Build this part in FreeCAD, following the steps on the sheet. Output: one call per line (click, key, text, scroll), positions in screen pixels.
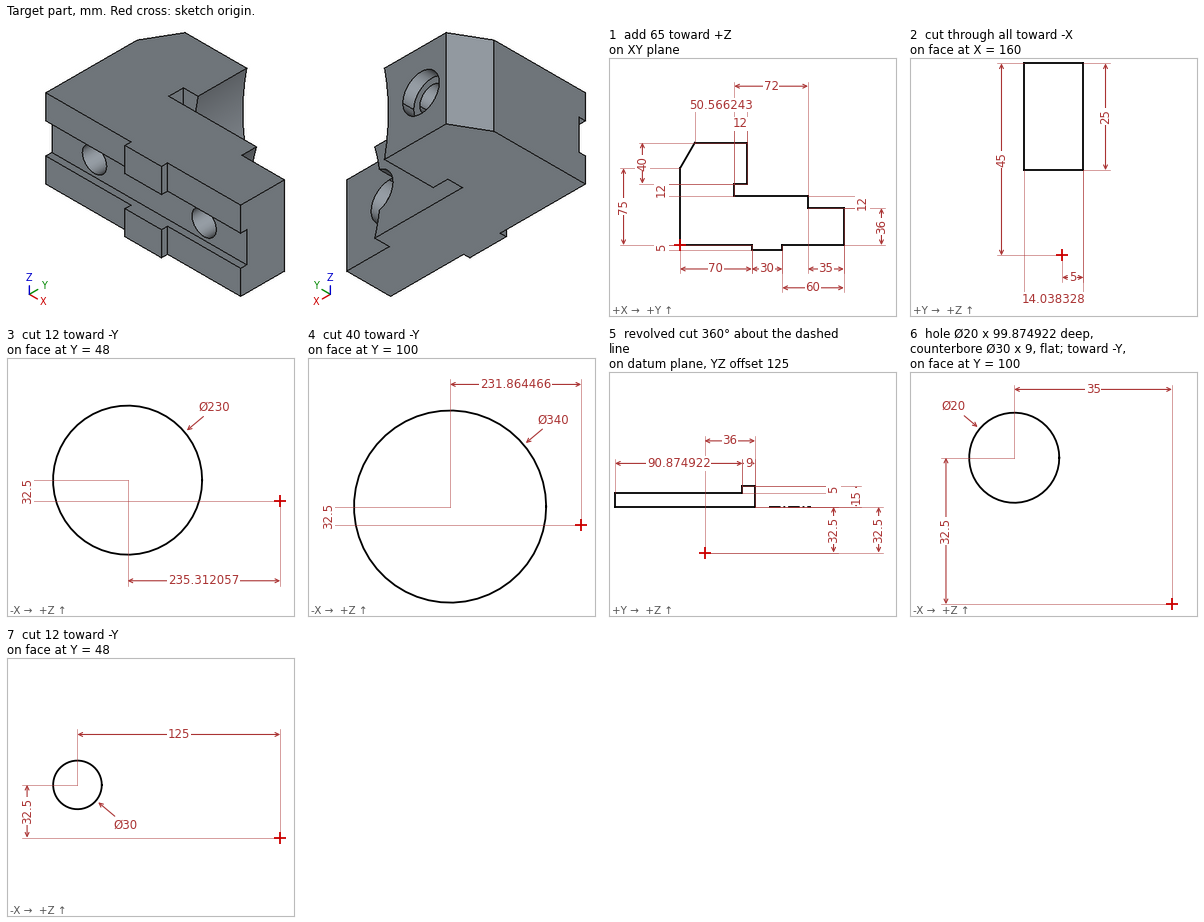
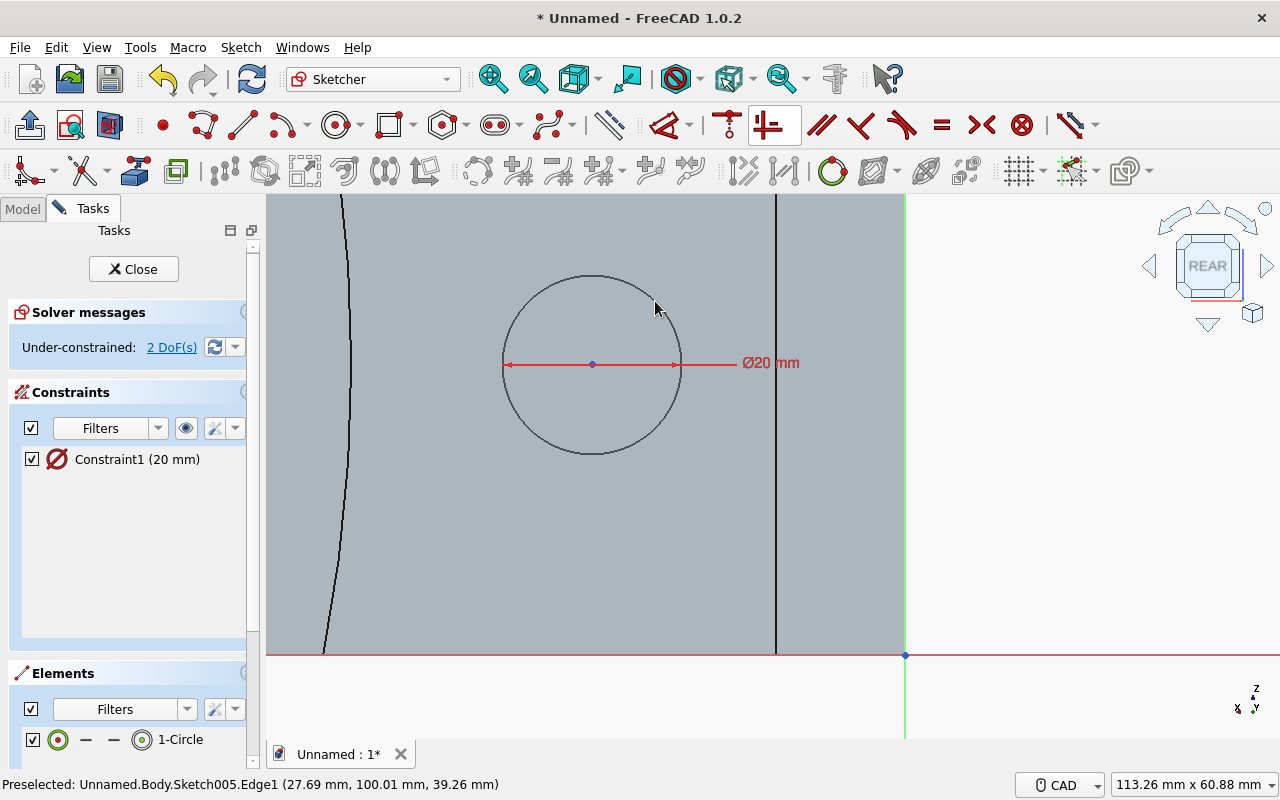
key(d)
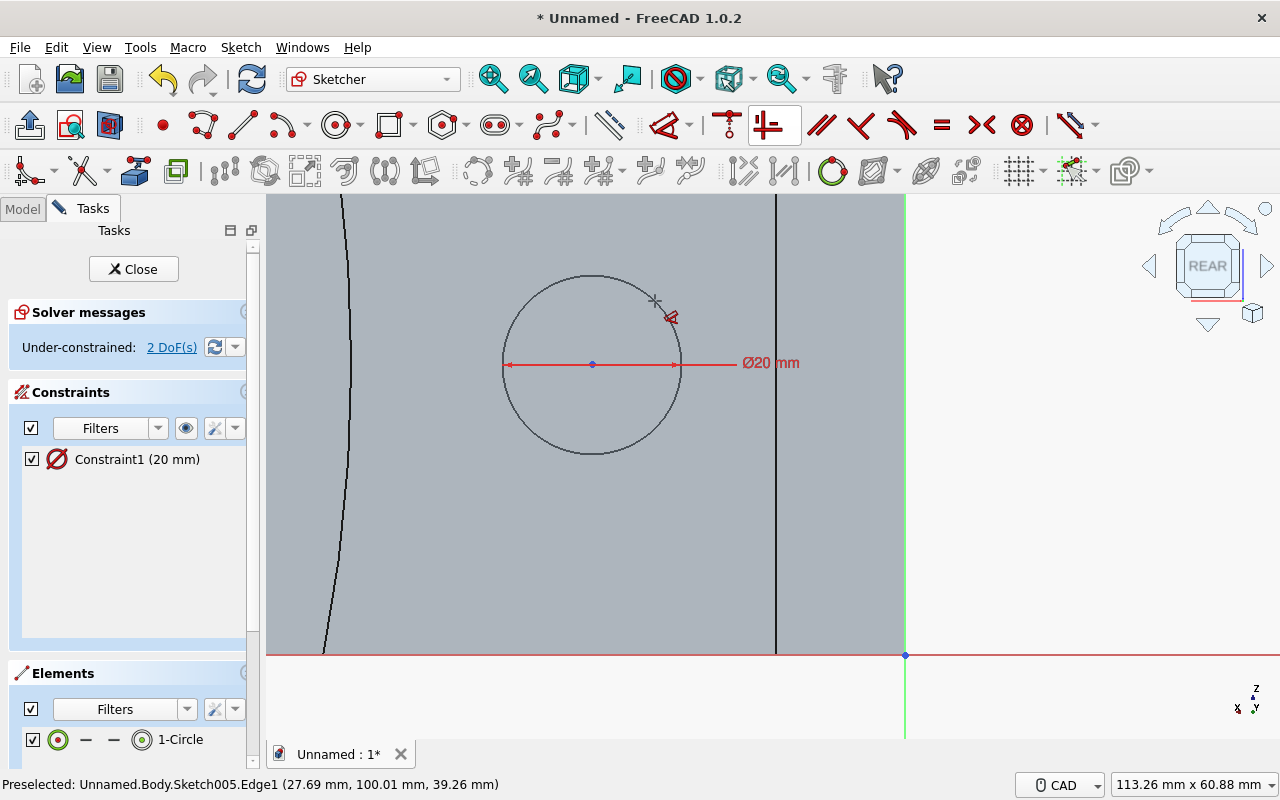
click(592, 365)
click(749, 689)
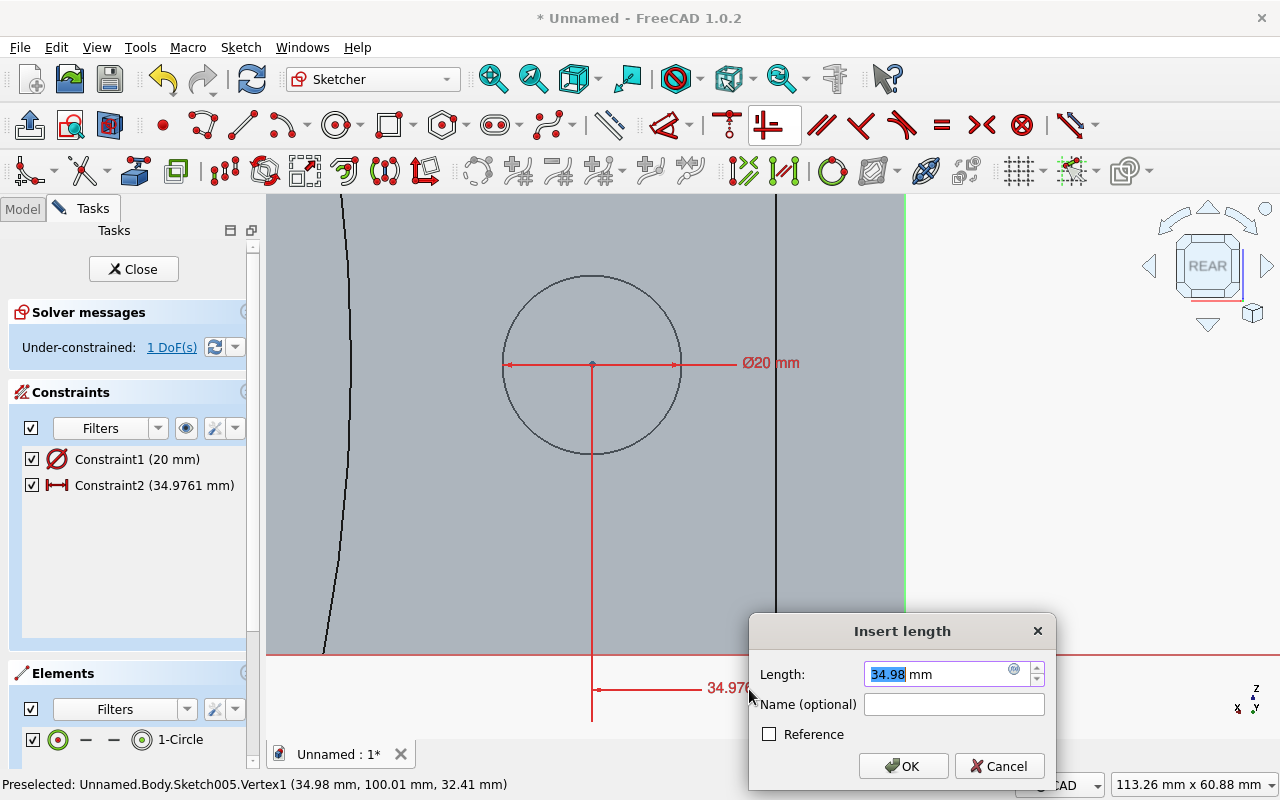
text(35)
key(Return)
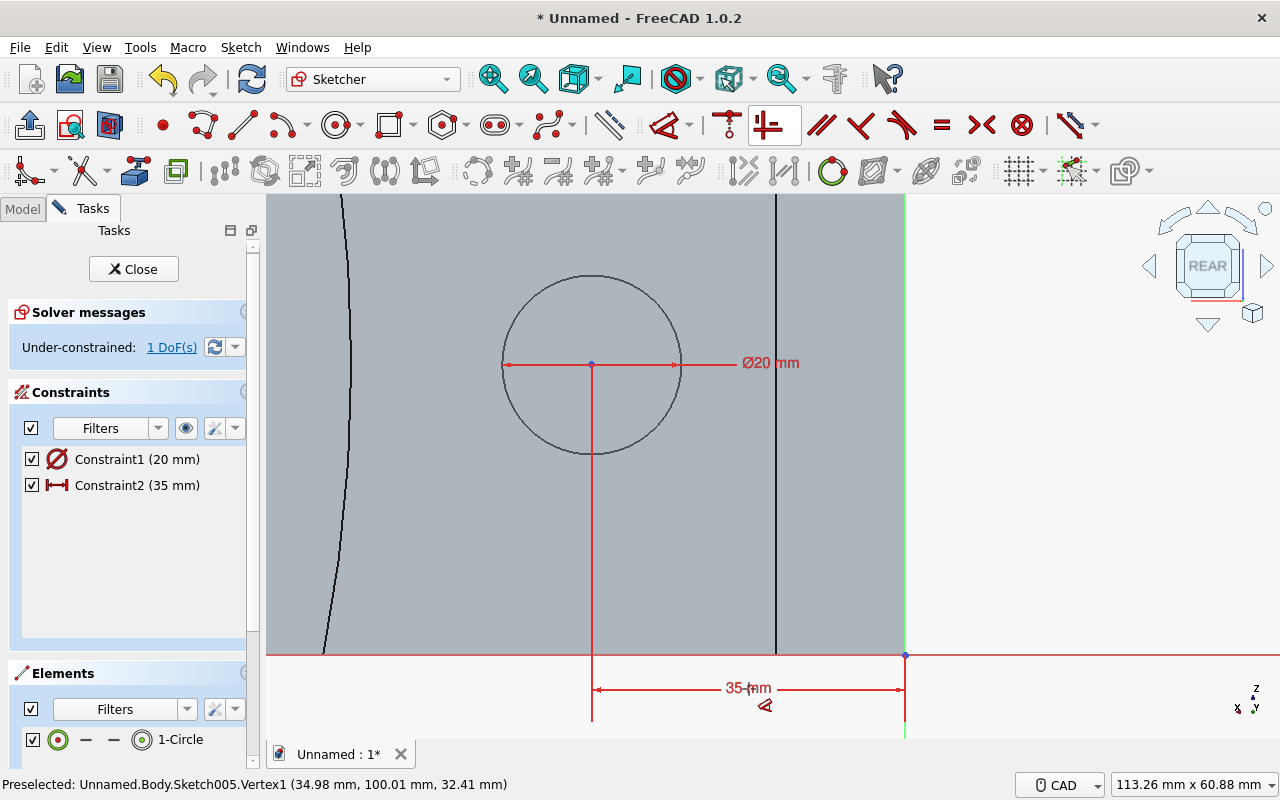
click(592, 365)
click(939, 510)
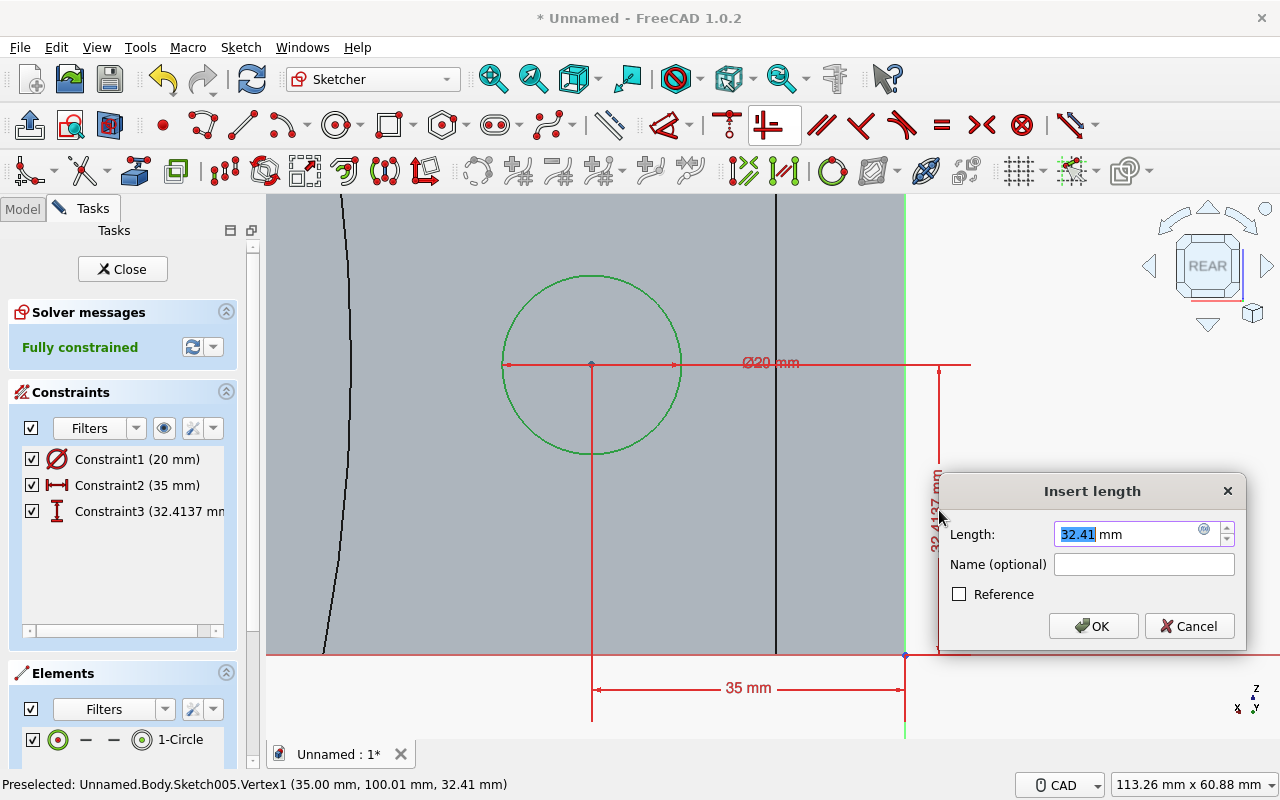
text(32.5)
key(Return)
key(Escape)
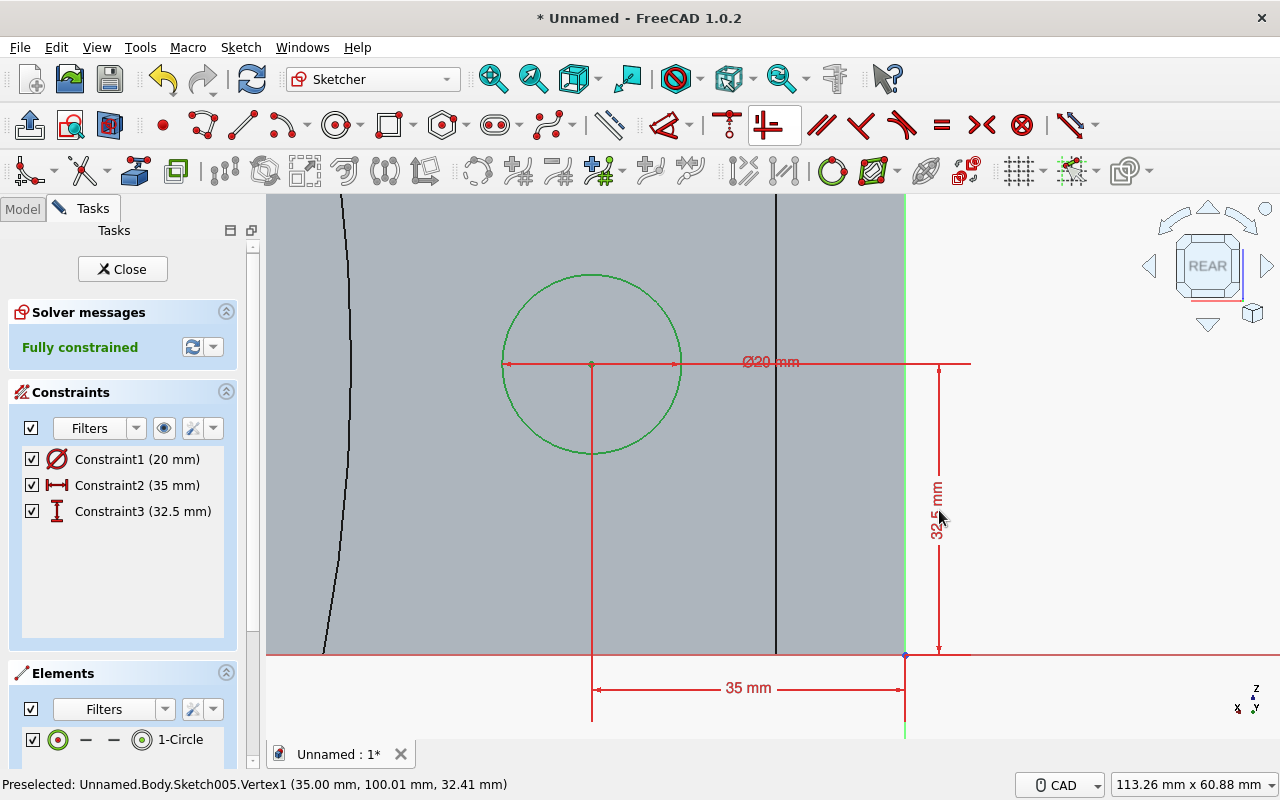
click(123, 269)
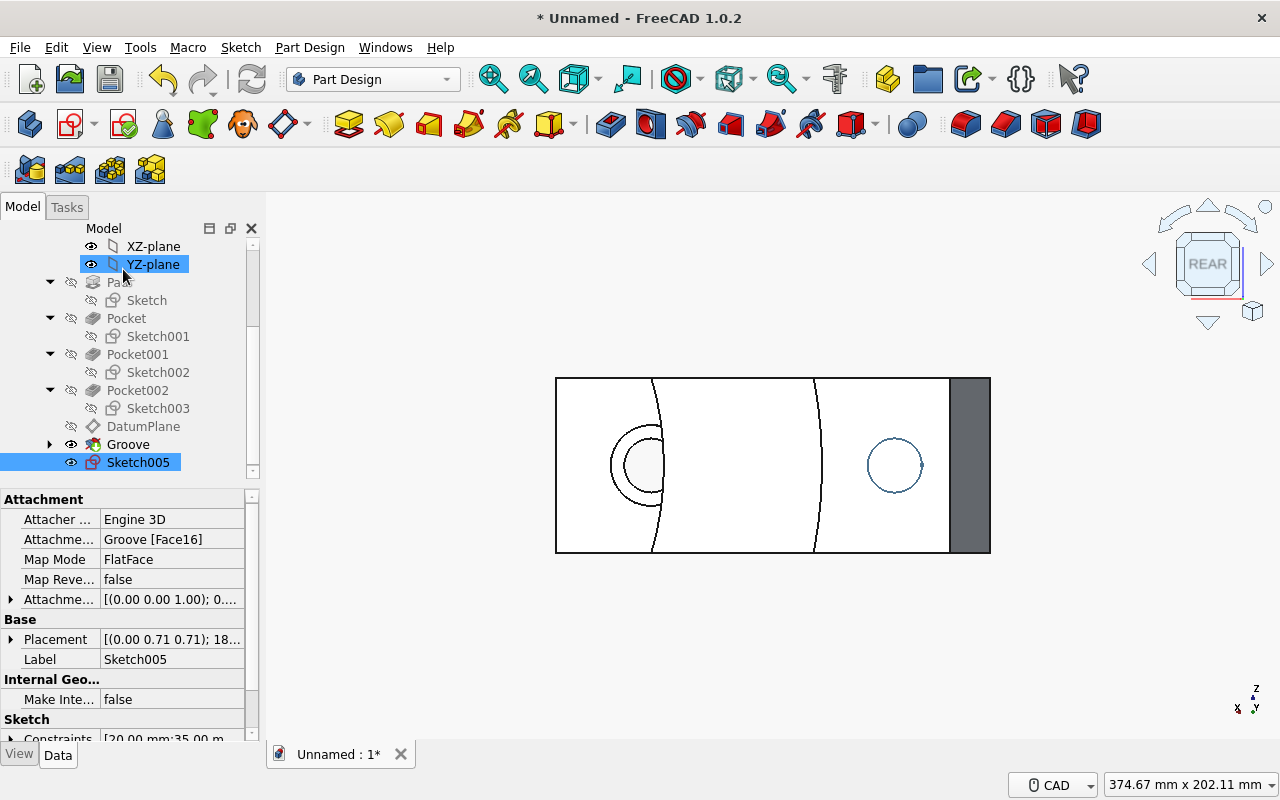
click(652, 124)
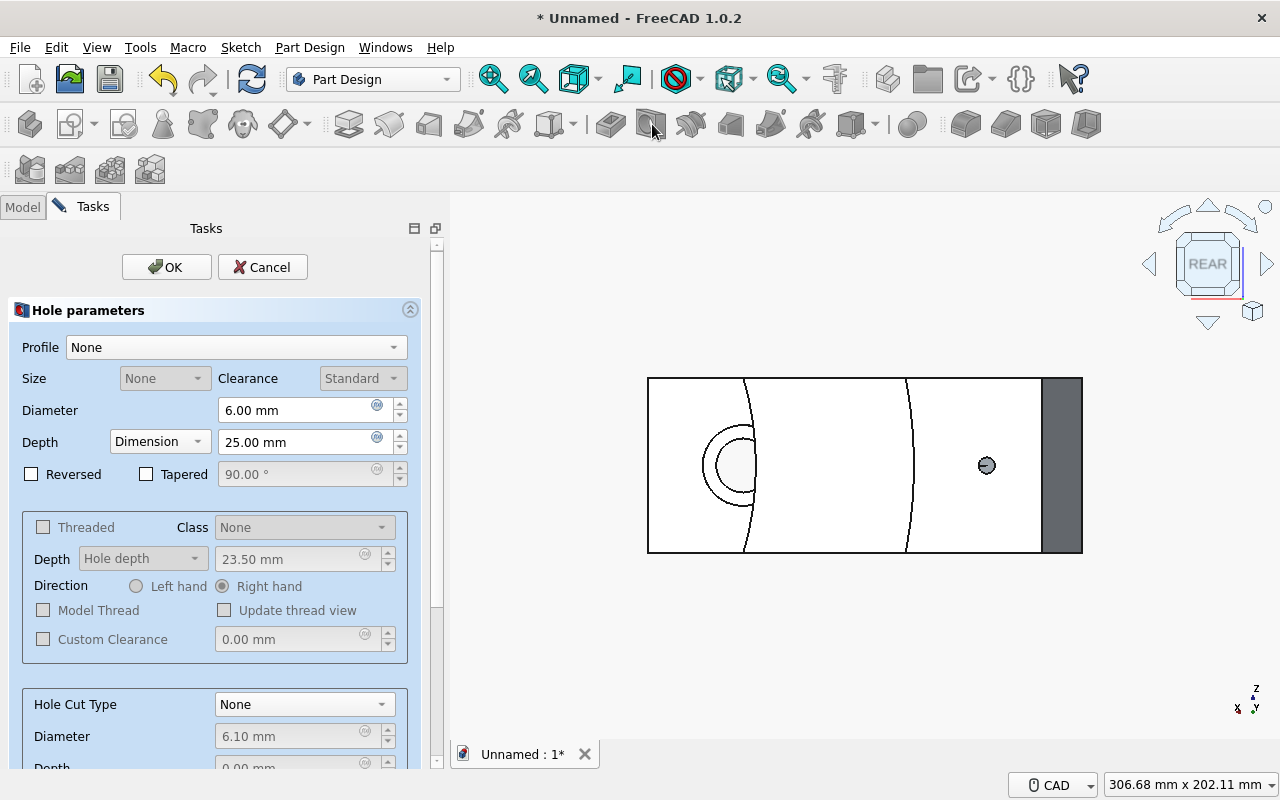
triple_click(305, 410)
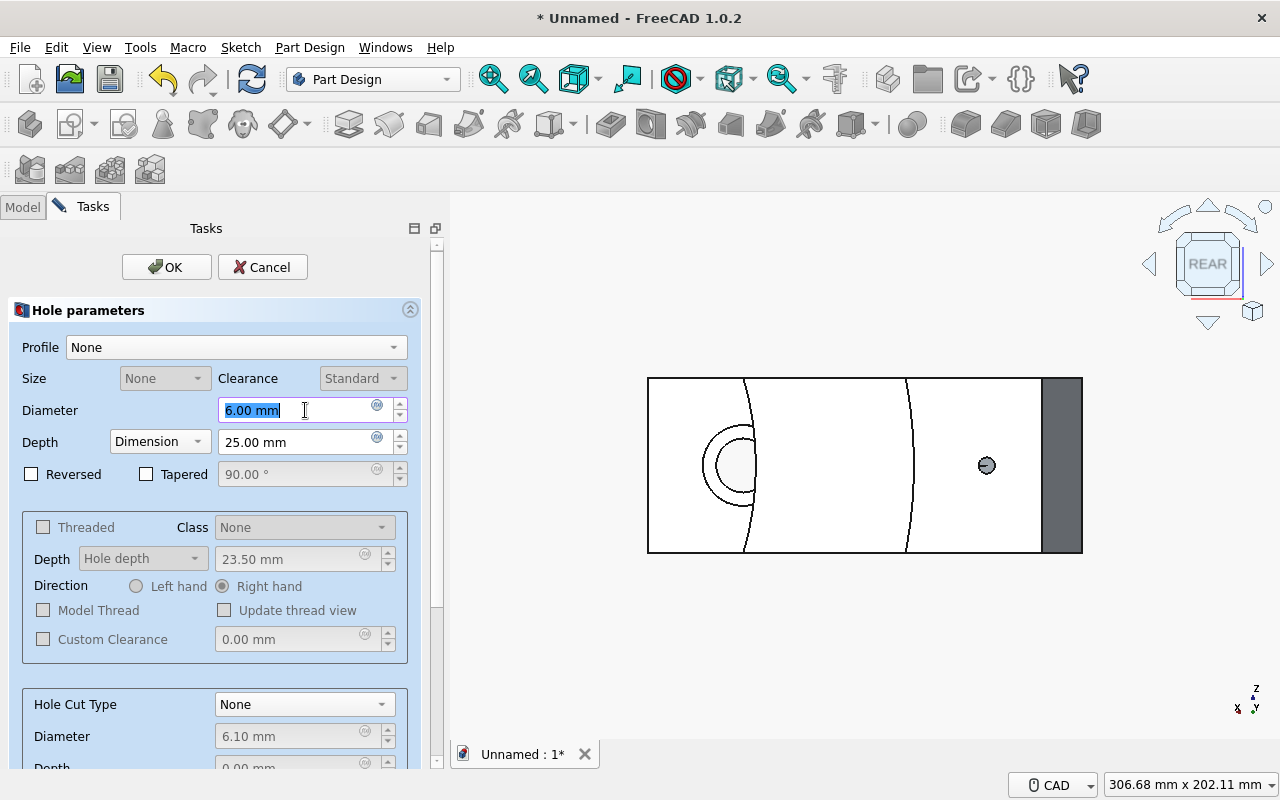
text(20)
key(Tab)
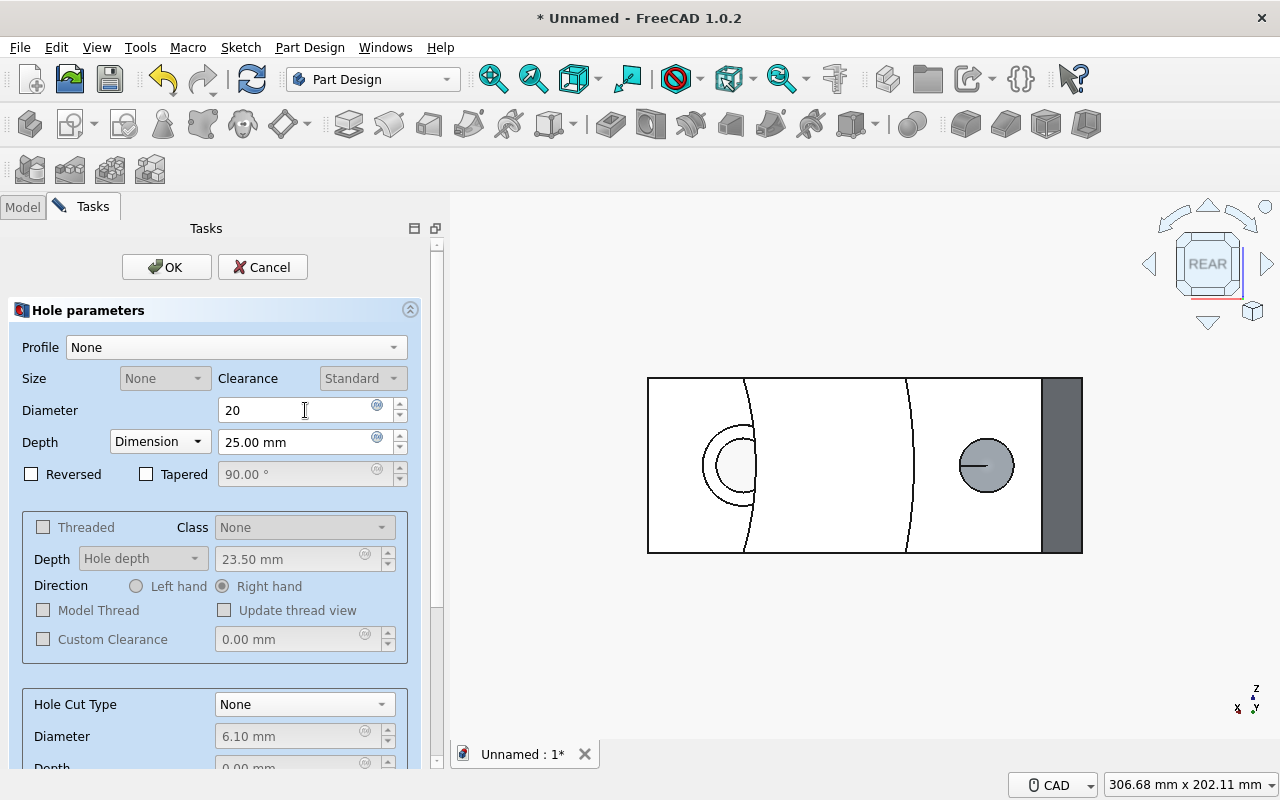
triple_click(305, 442)